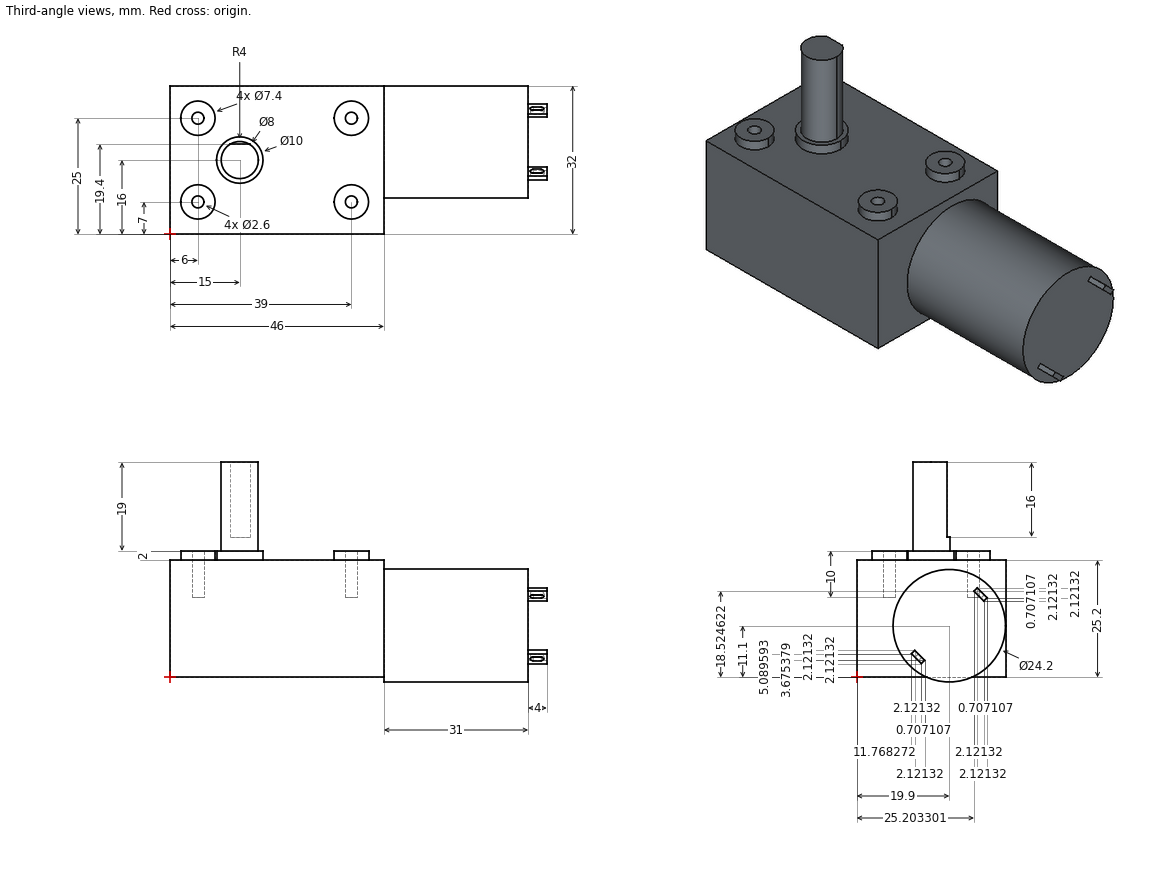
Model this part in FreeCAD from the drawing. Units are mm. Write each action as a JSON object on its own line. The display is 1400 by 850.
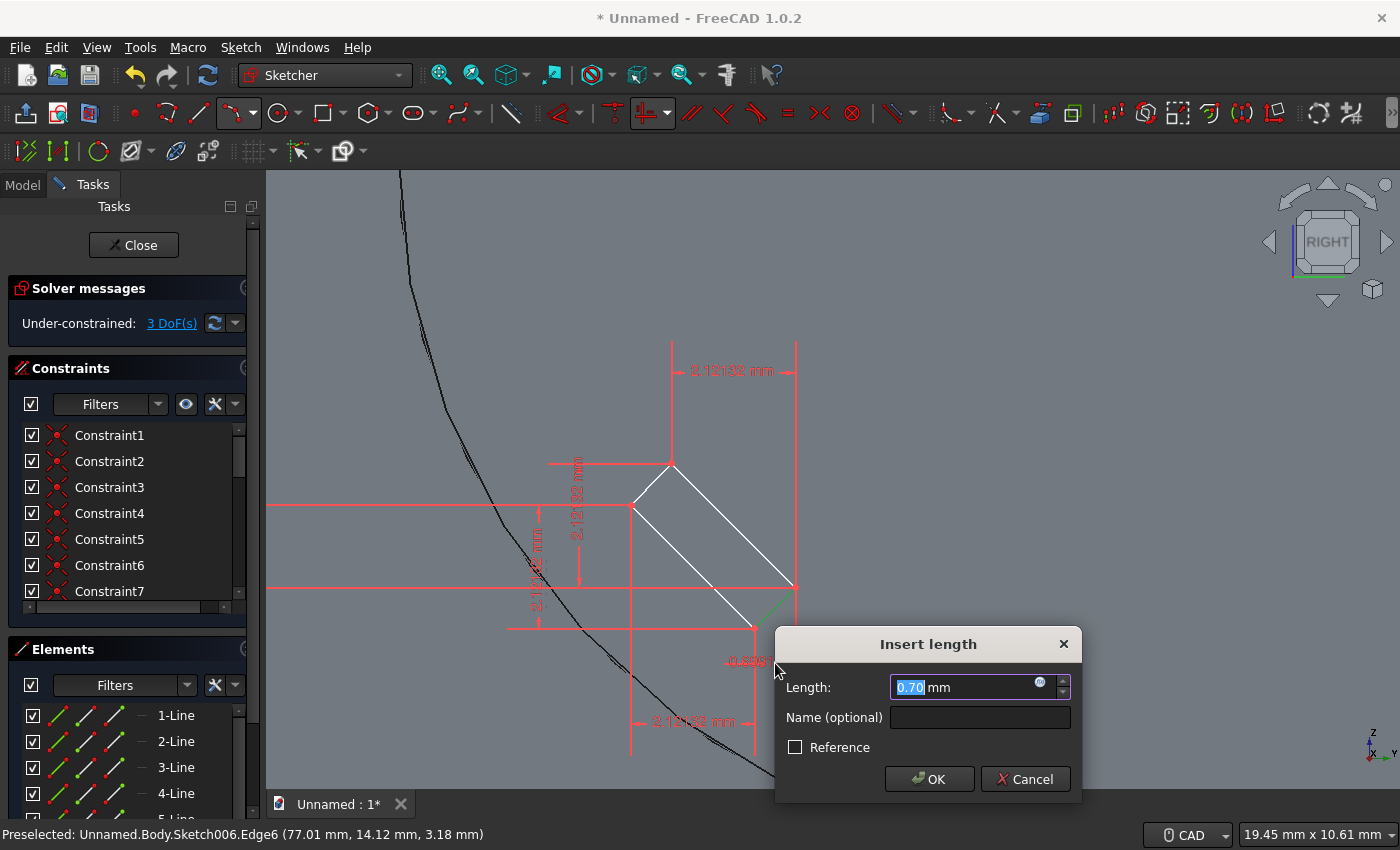
{"action": "type", "text": "0.707107"}
{"action": "key", "text": "Return"}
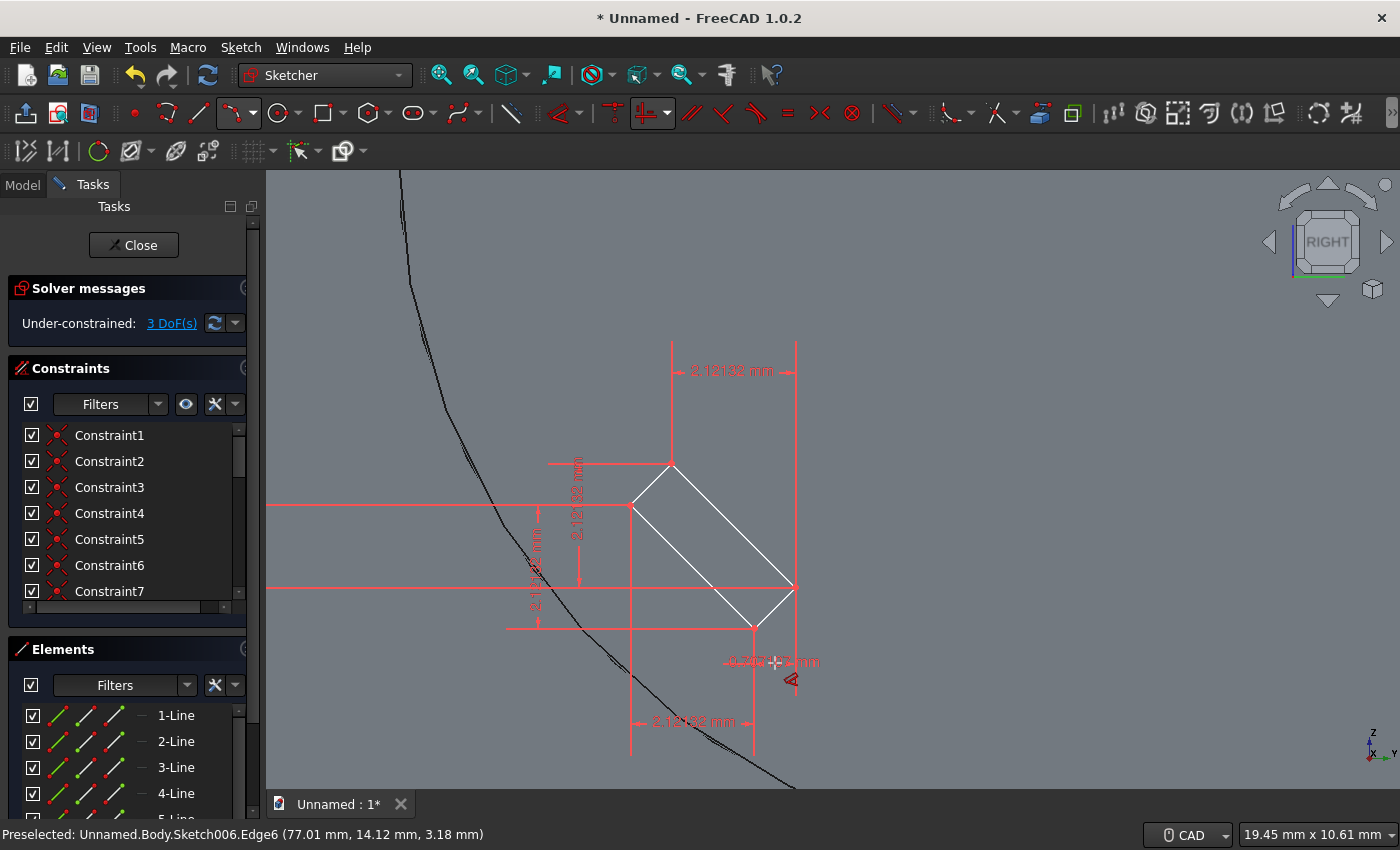
{"action": "scroll", "coordinate": [767, 618], "scroll_direction": "down", "scroll_amount": 5}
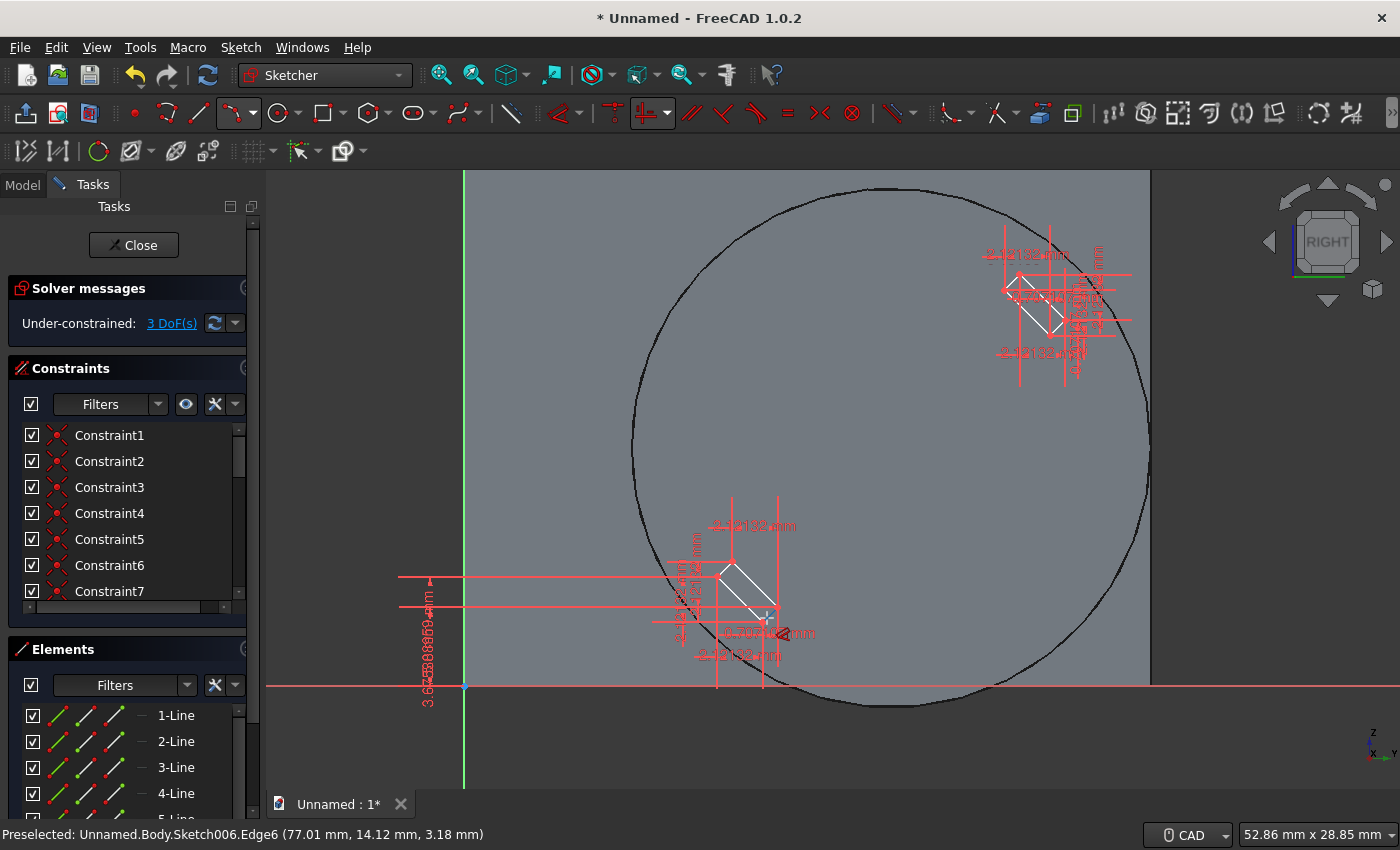
{"action": "left_click", "coordinate": [1005, 290]}
{"action": "left_click", "coordinate": [735, 720]}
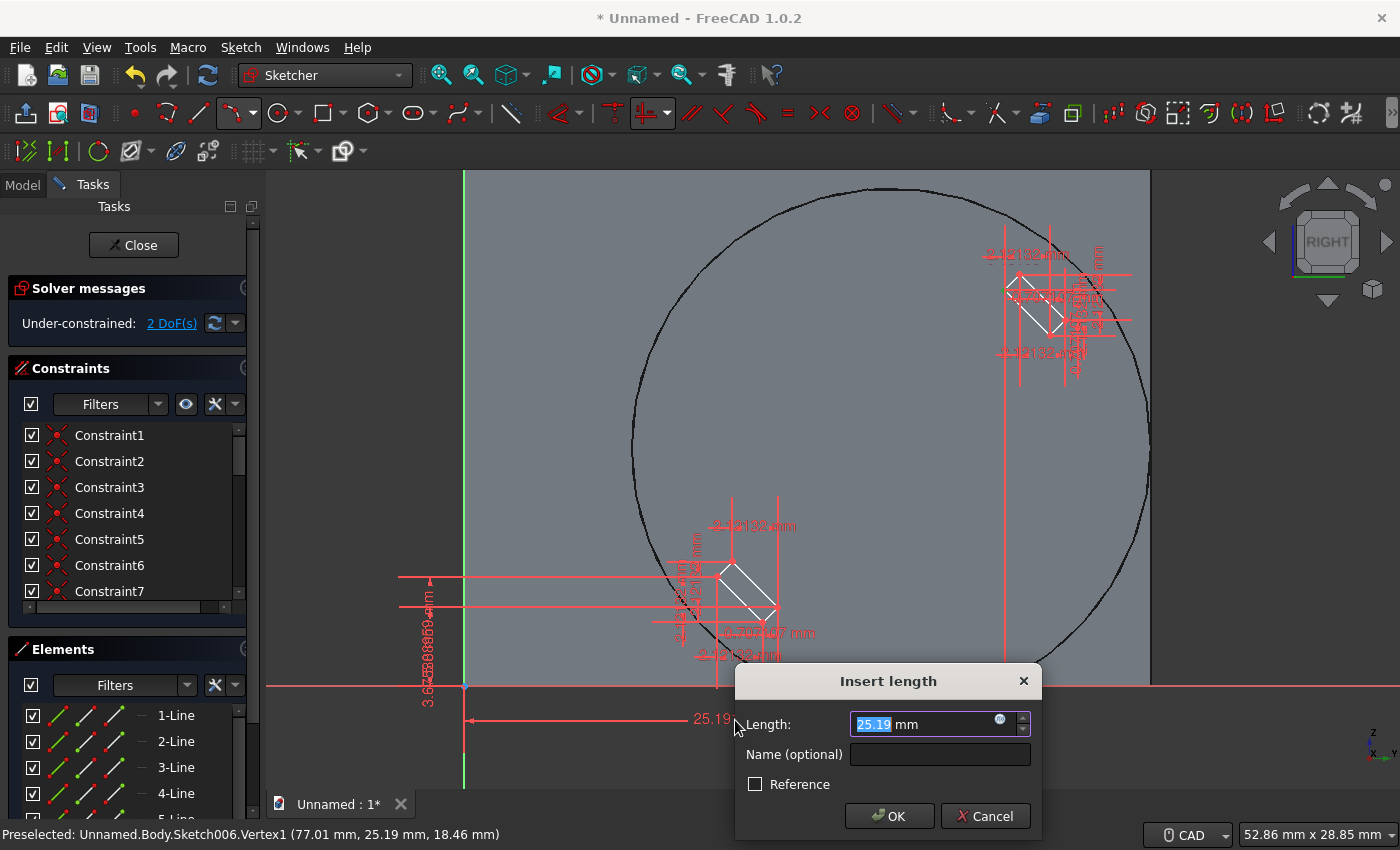
{"action": "type", "text": "25.203301"}
{"action": "key", "text": "Return"}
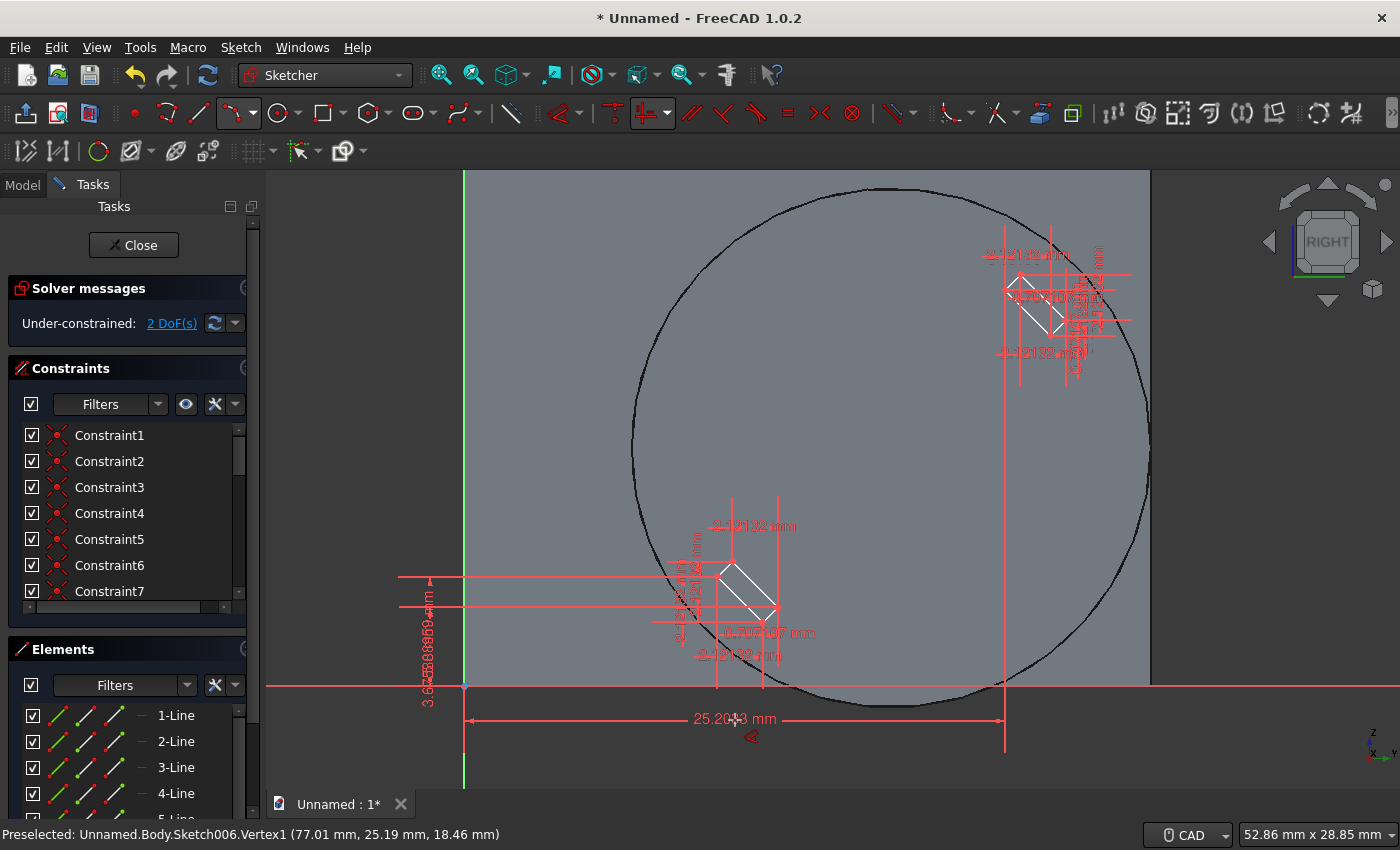
{"action": "left_click", "coordinate": [1005, 290]}
{"action": "left_click", "coordinate": [430, 488]}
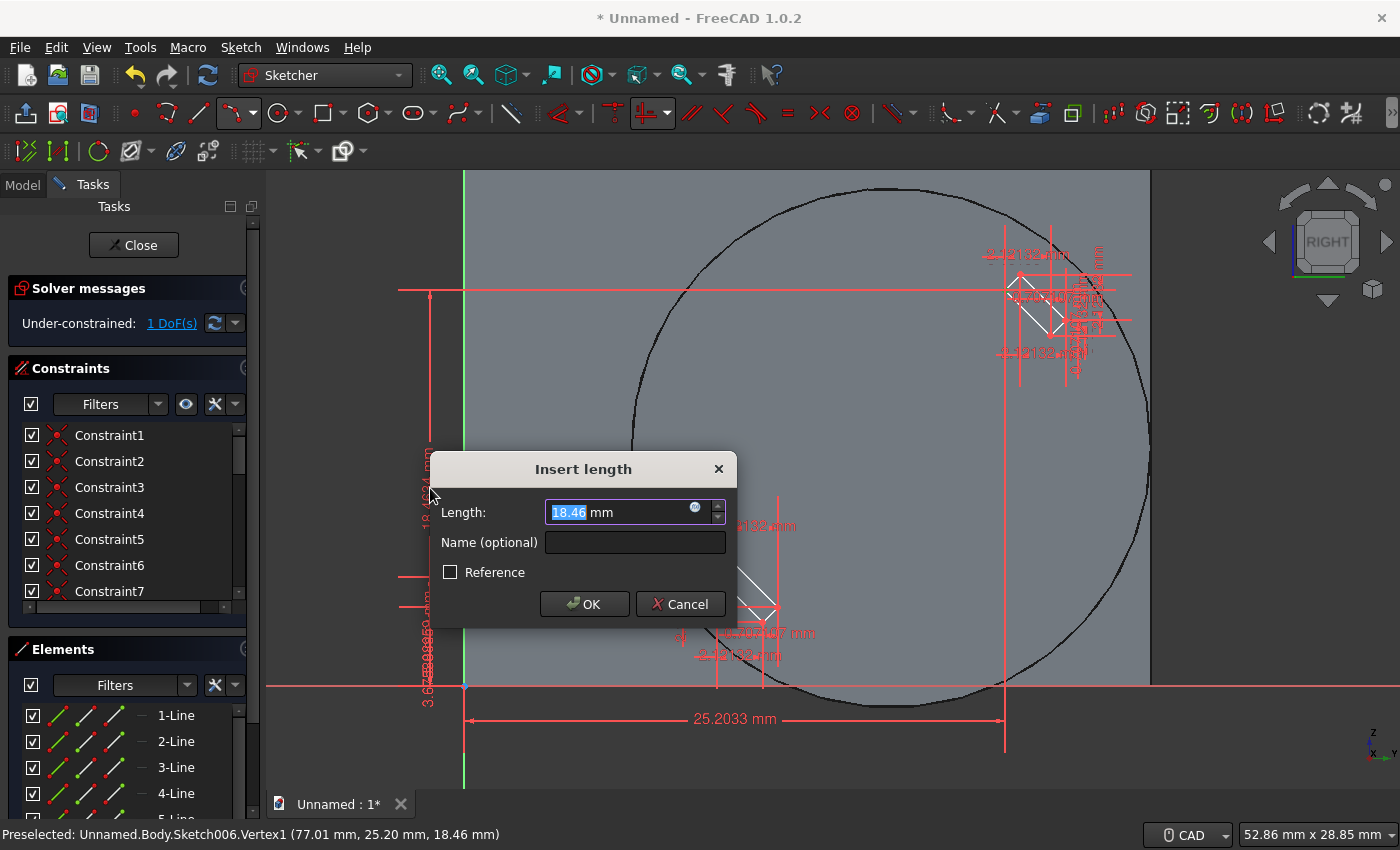
{"action": "type", "text": "18.524622"}
{"action": "key", "text": "Return"}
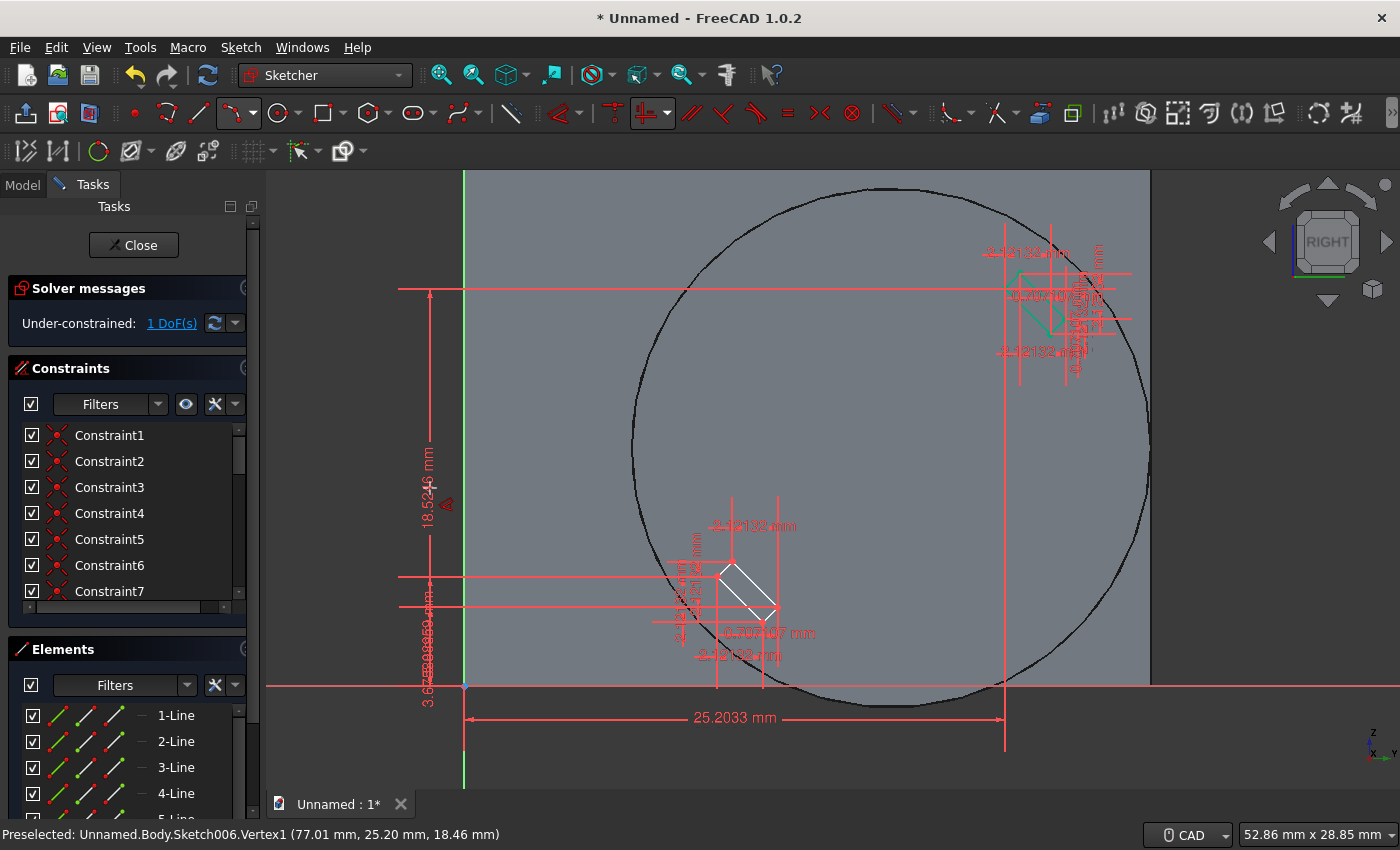
{"action": "left_click", "coordinate": [717, 577]}
{"action": "left_click", "coordinate": [591, 720]}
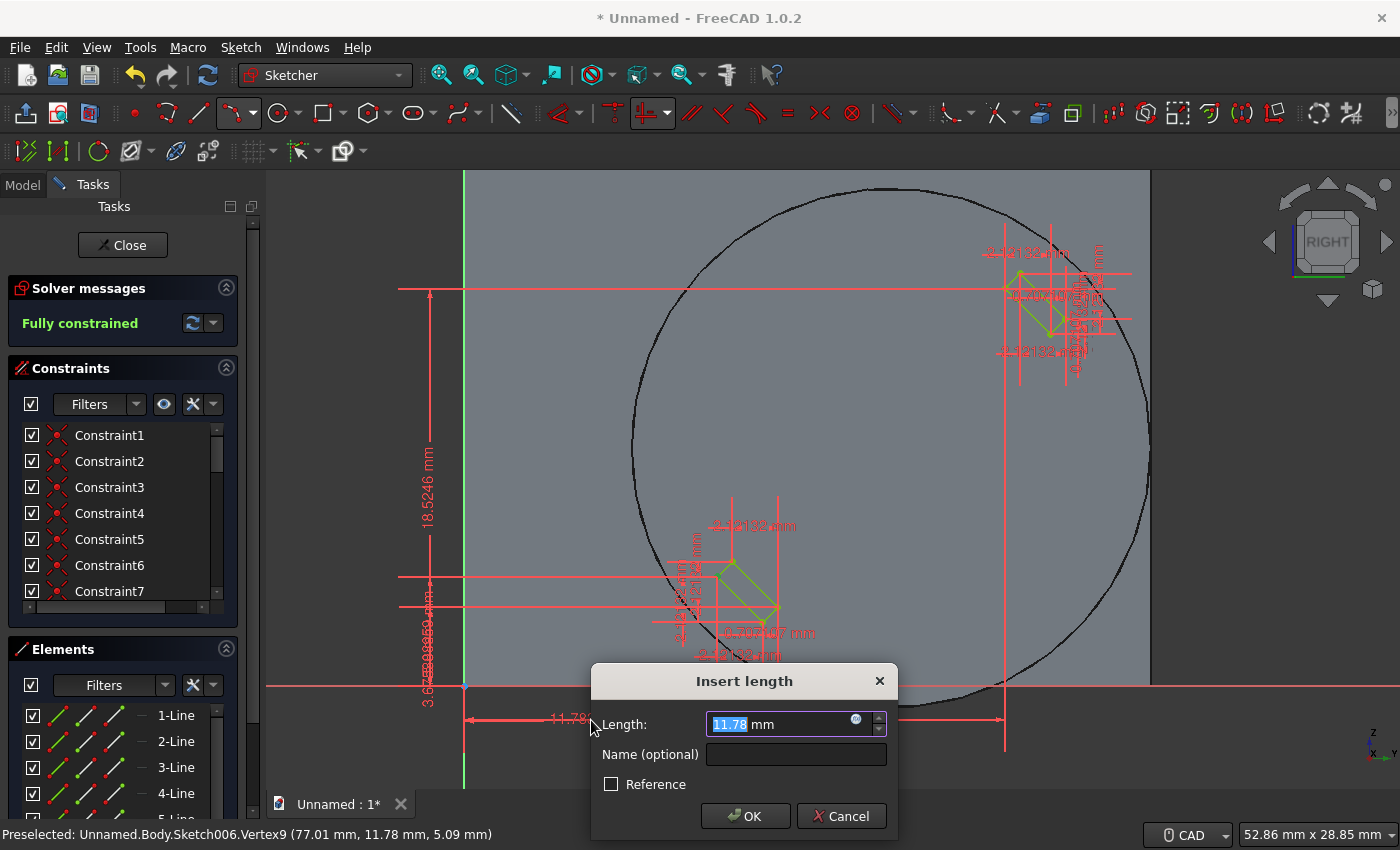
{"action": "type", "text": "11.768272"}
{"action": "key", "text": "Return"}
{"action": "key", "text": "Escape"}